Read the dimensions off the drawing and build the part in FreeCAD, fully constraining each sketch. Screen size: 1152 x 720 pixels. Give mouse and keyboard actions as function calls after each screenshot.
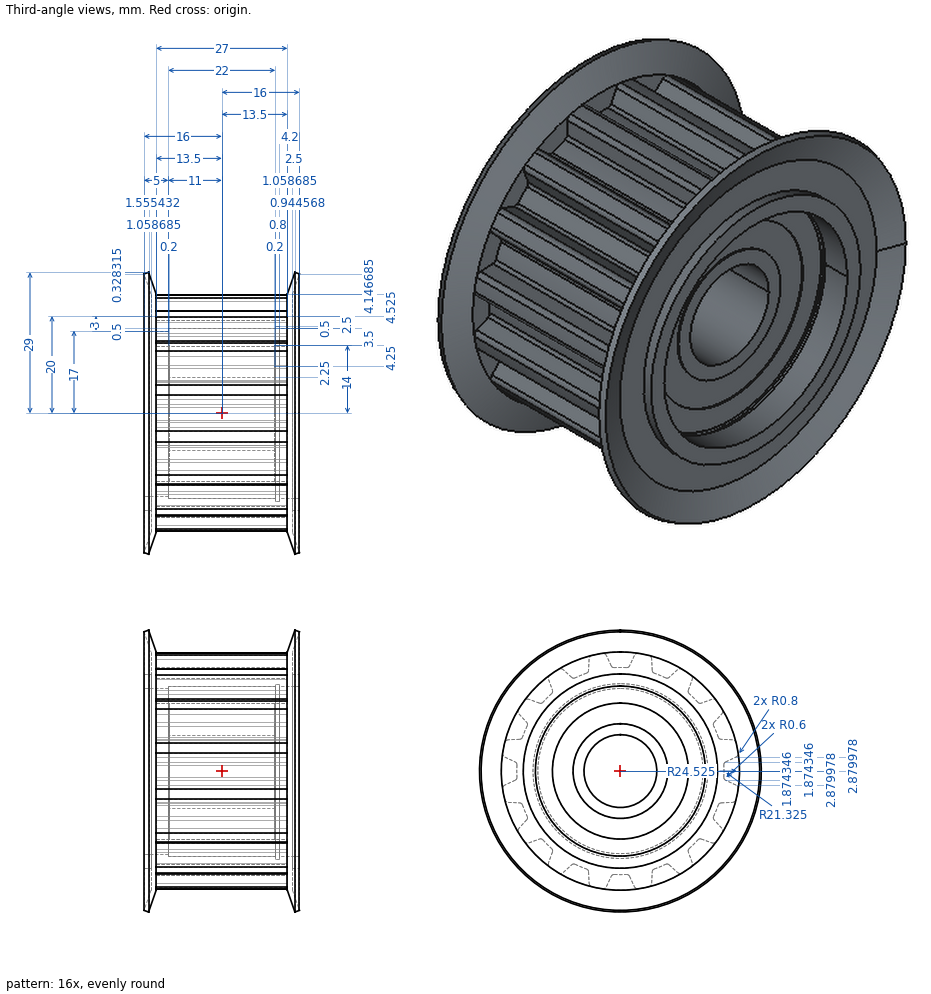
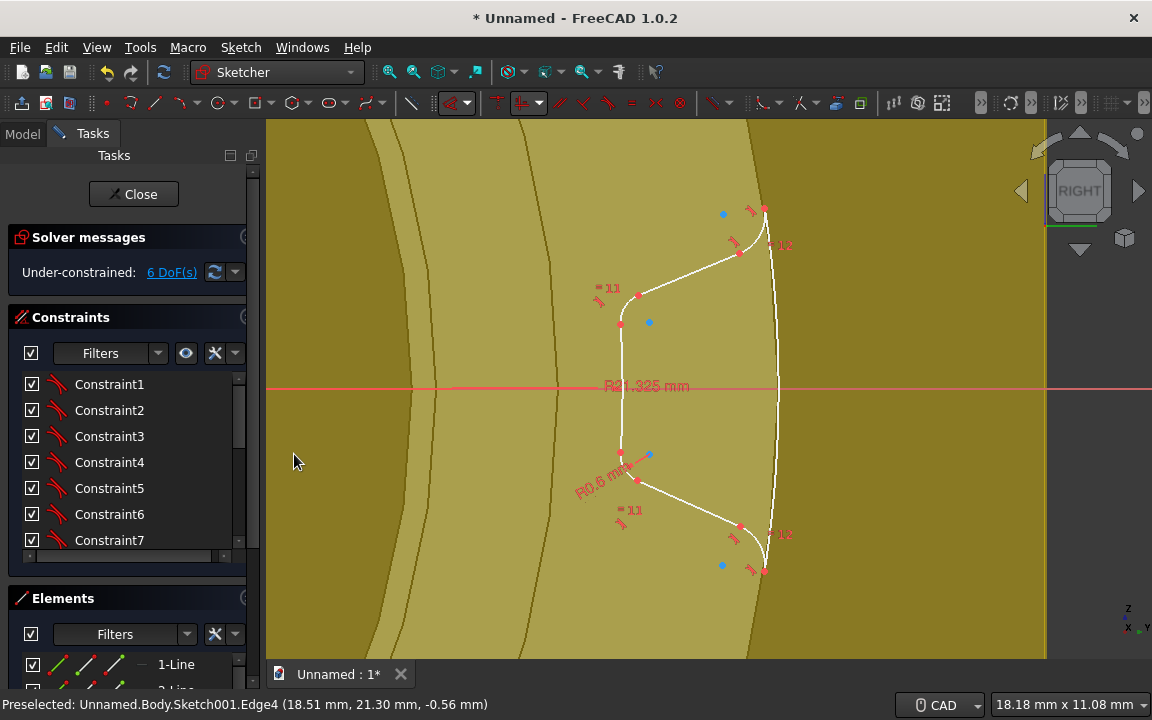
click(753, 244)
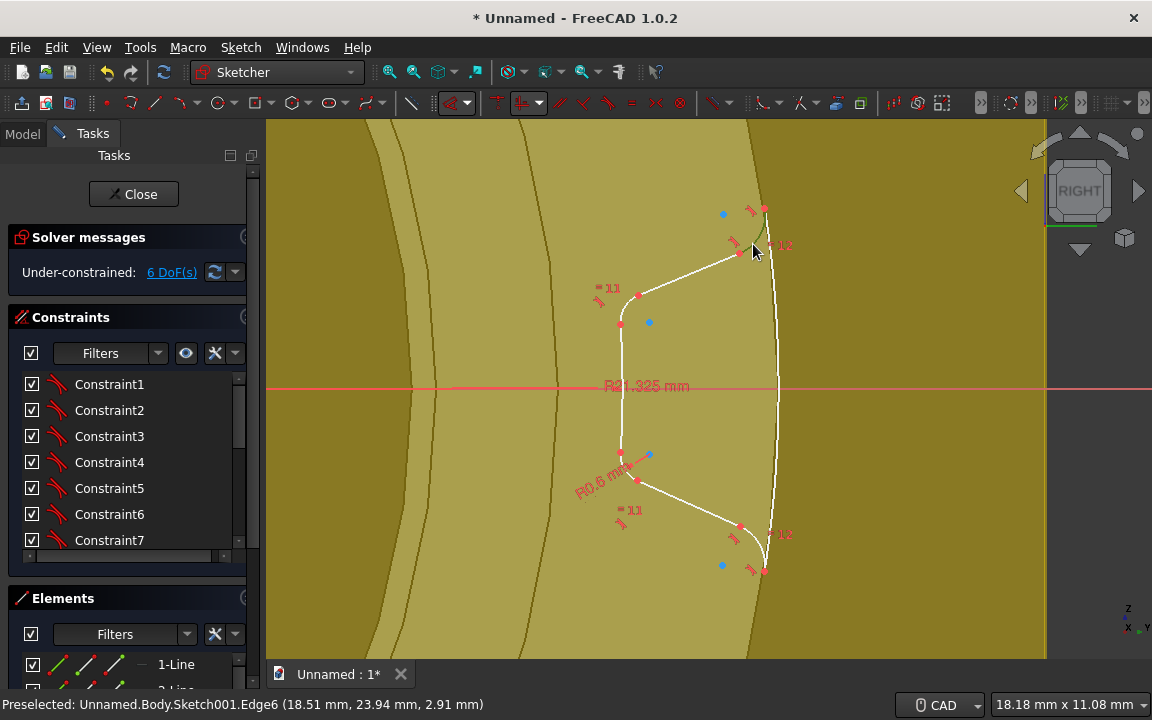
key(k)
key(r)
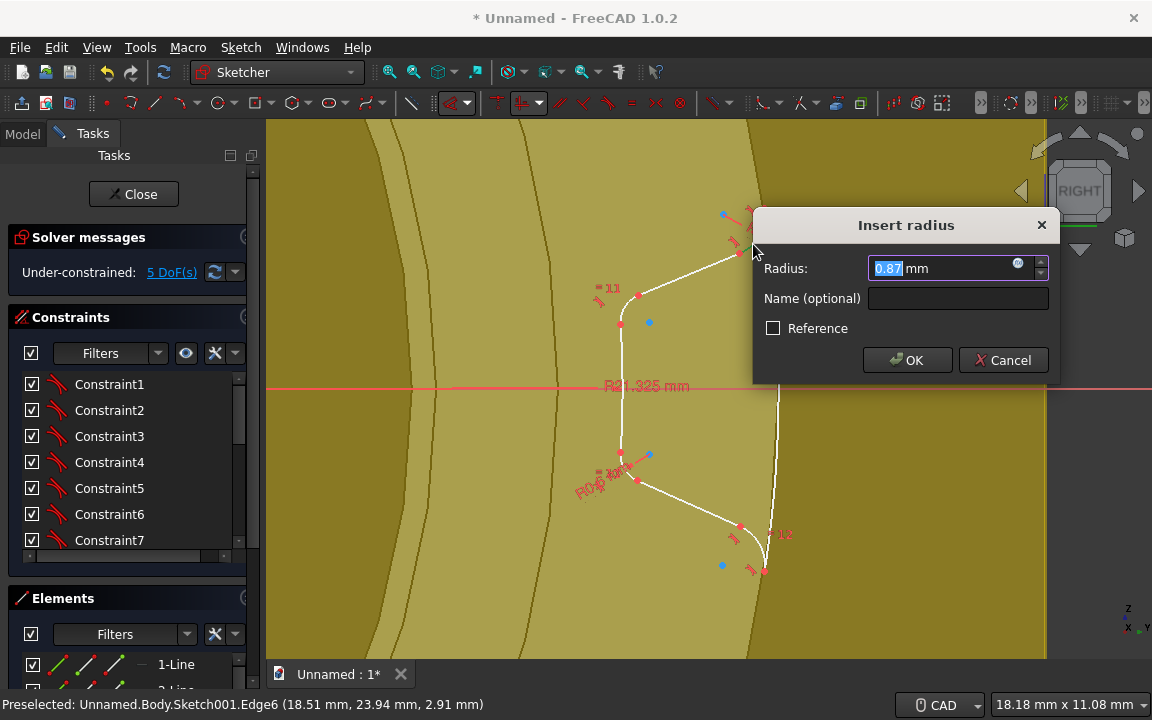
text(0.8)
key(Return)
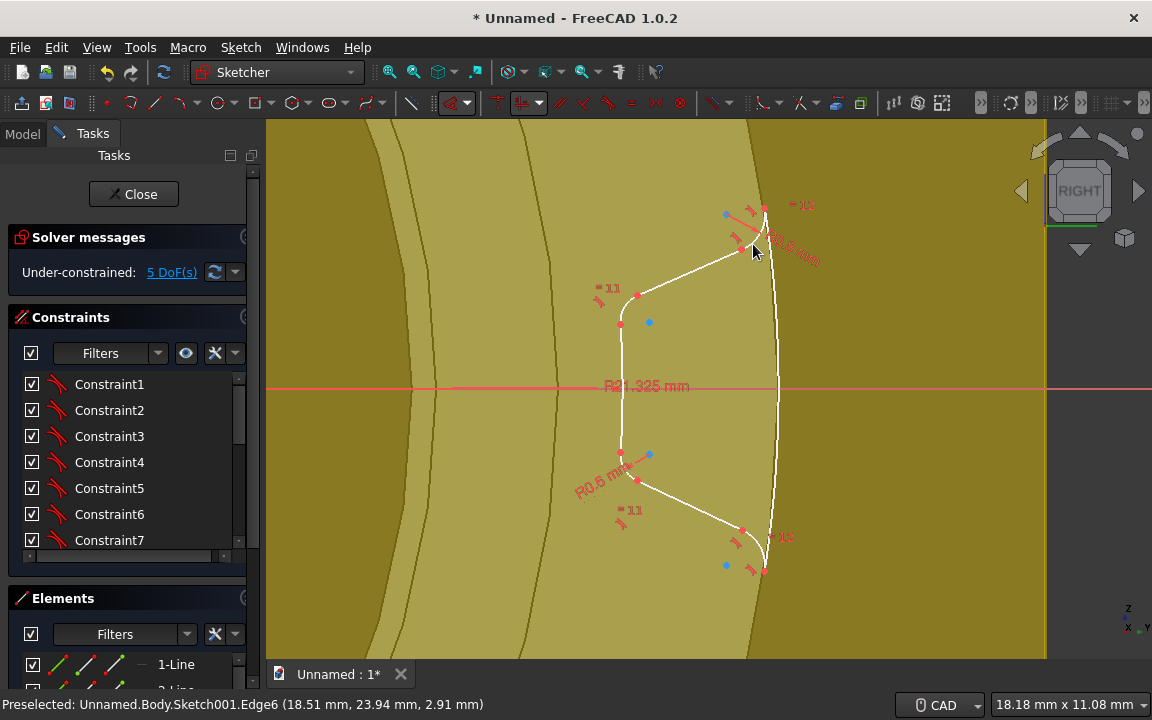
click(776, 463)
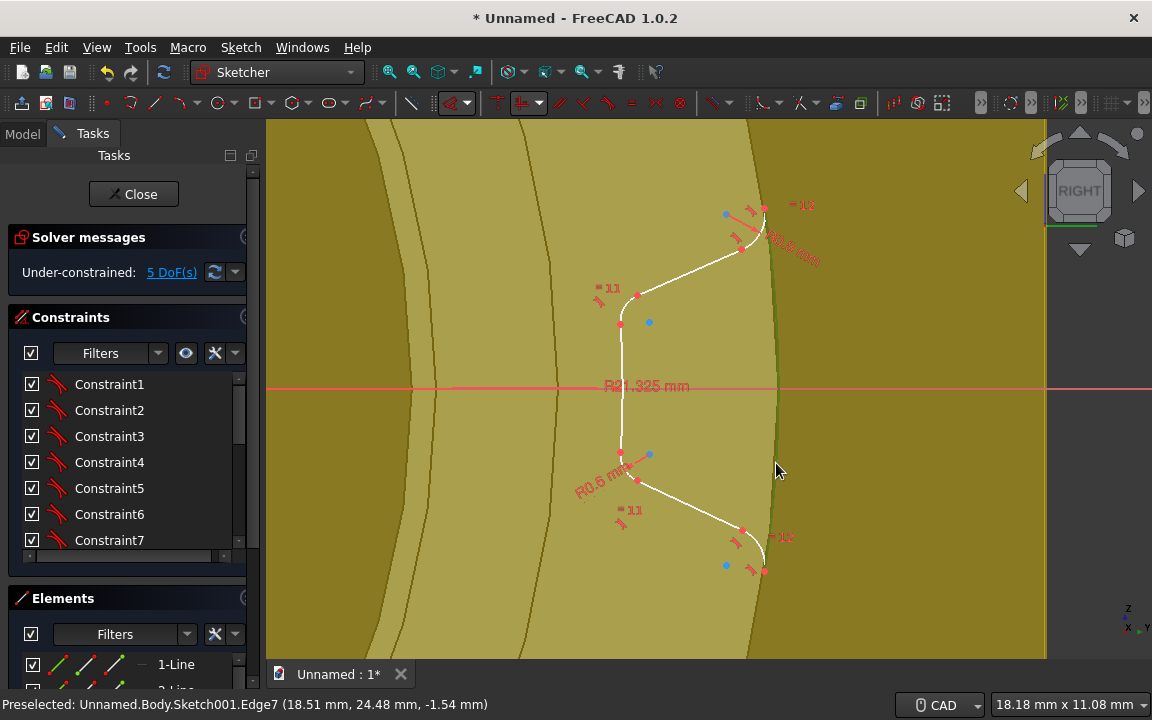
key(k)
key(r)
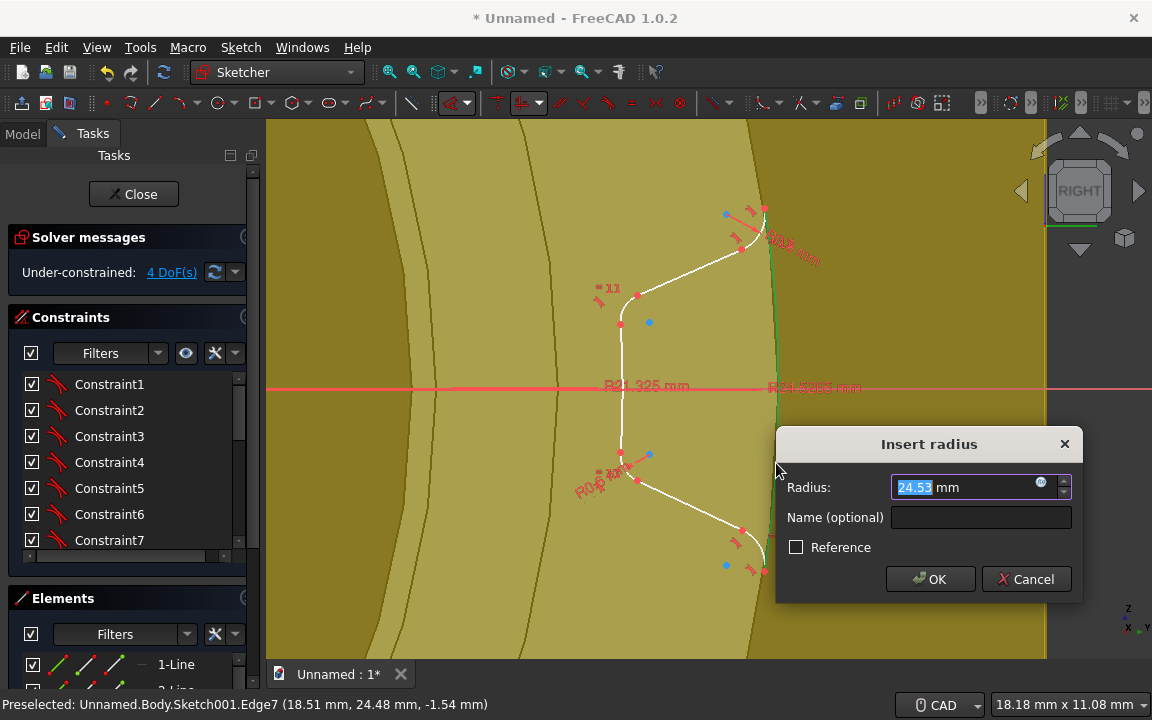
text(24.525)
key(Return)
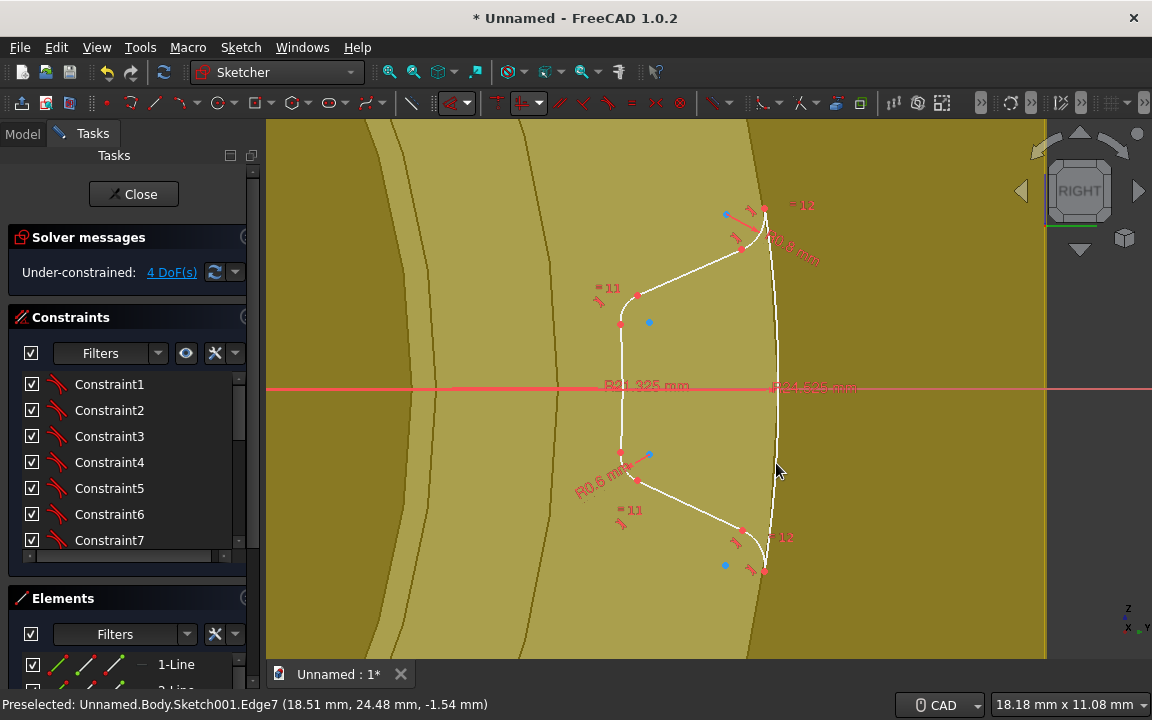
click(743, 530)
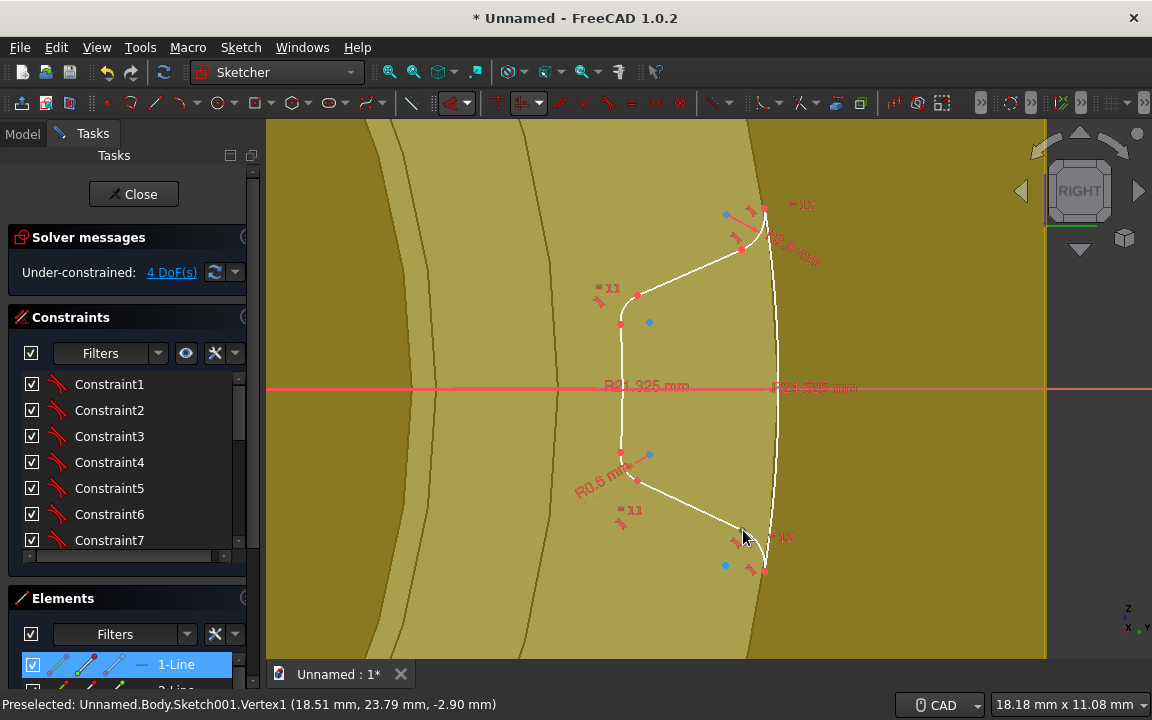
click(470, 104)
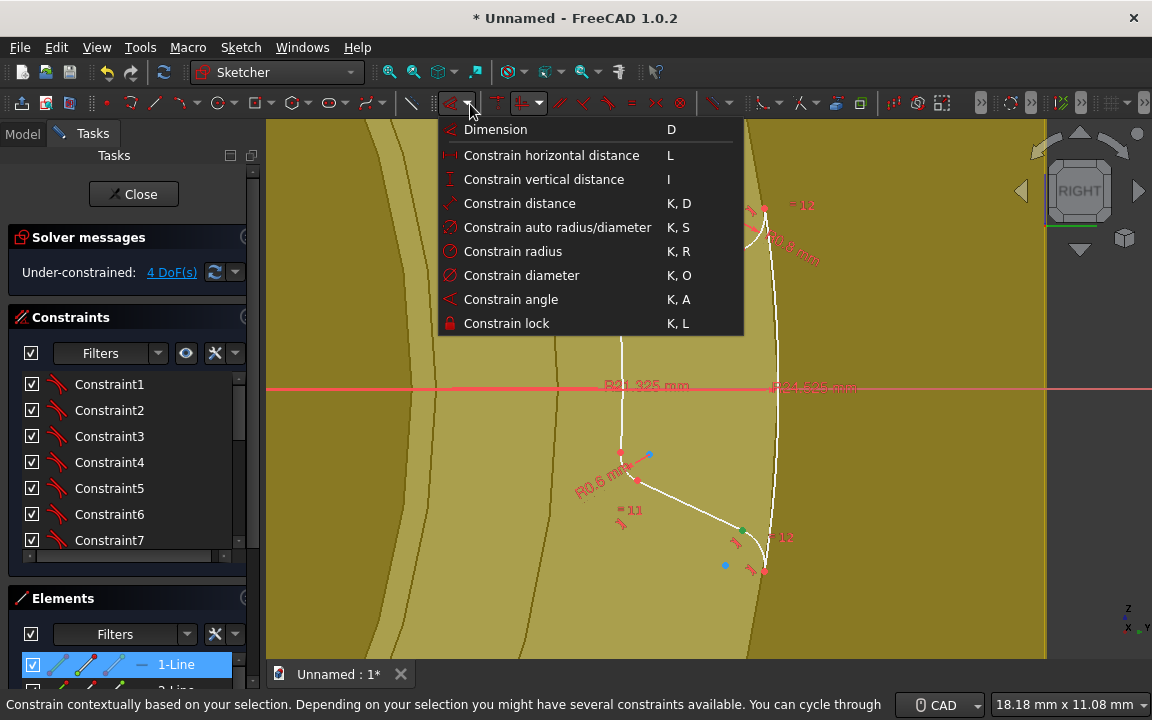
click(591, 179)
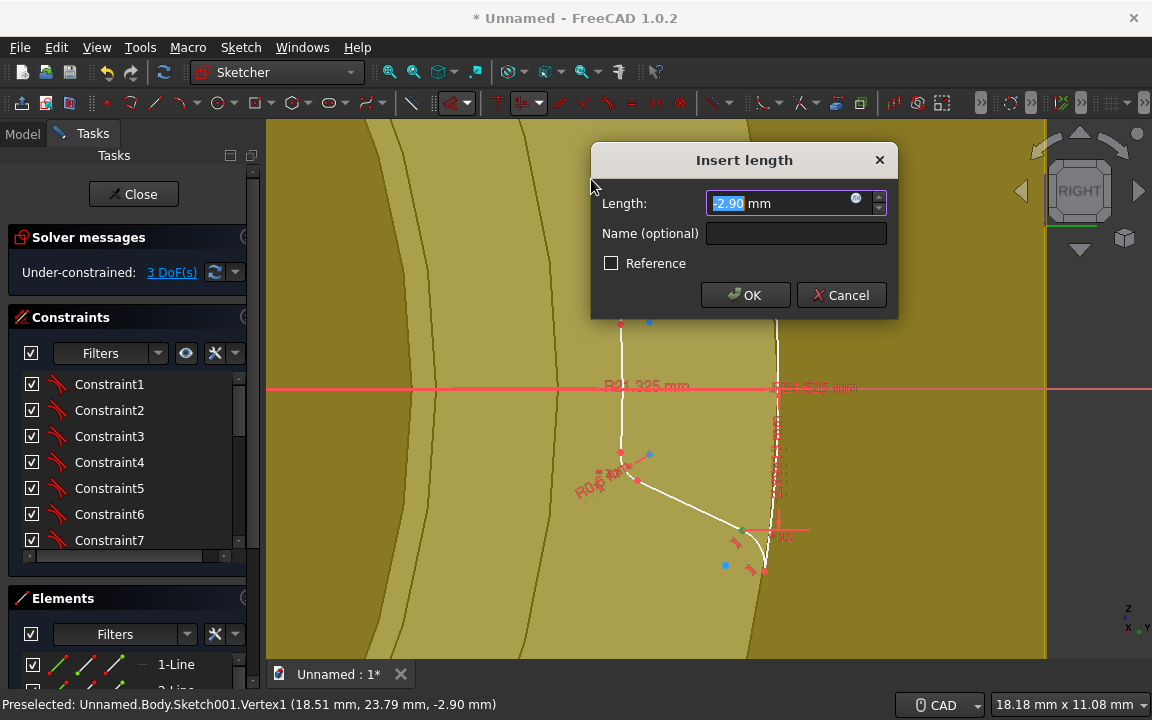
text(-2.879978)
key(Return)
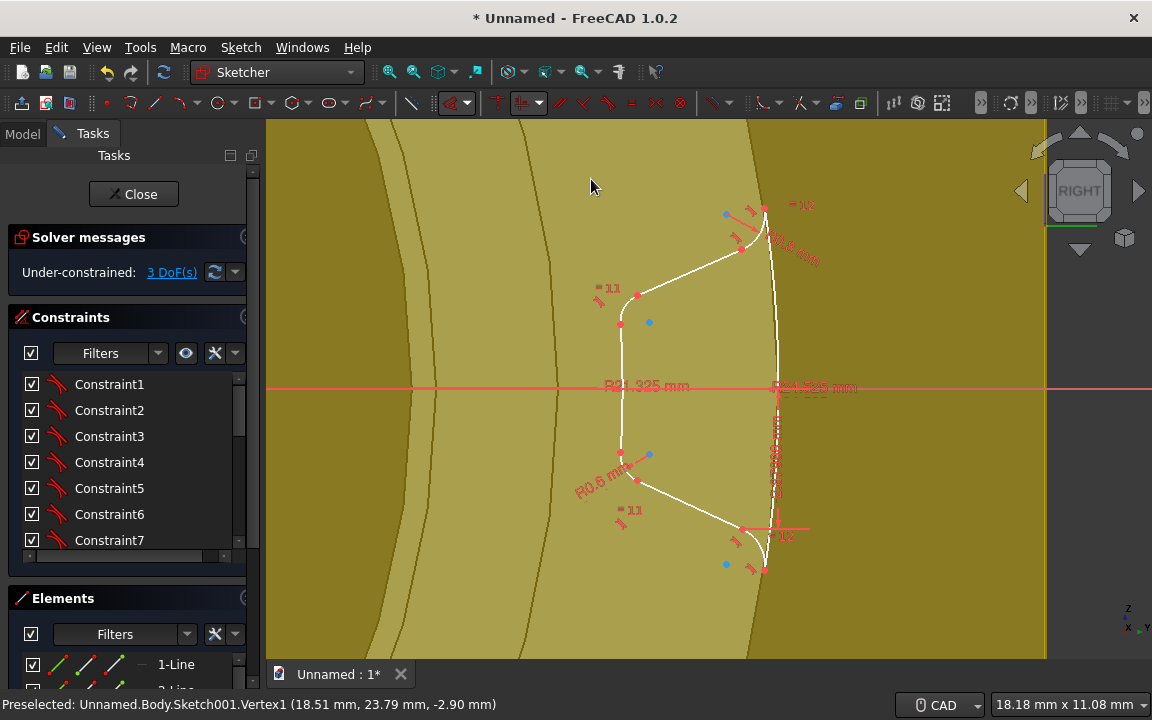
click(638, 481)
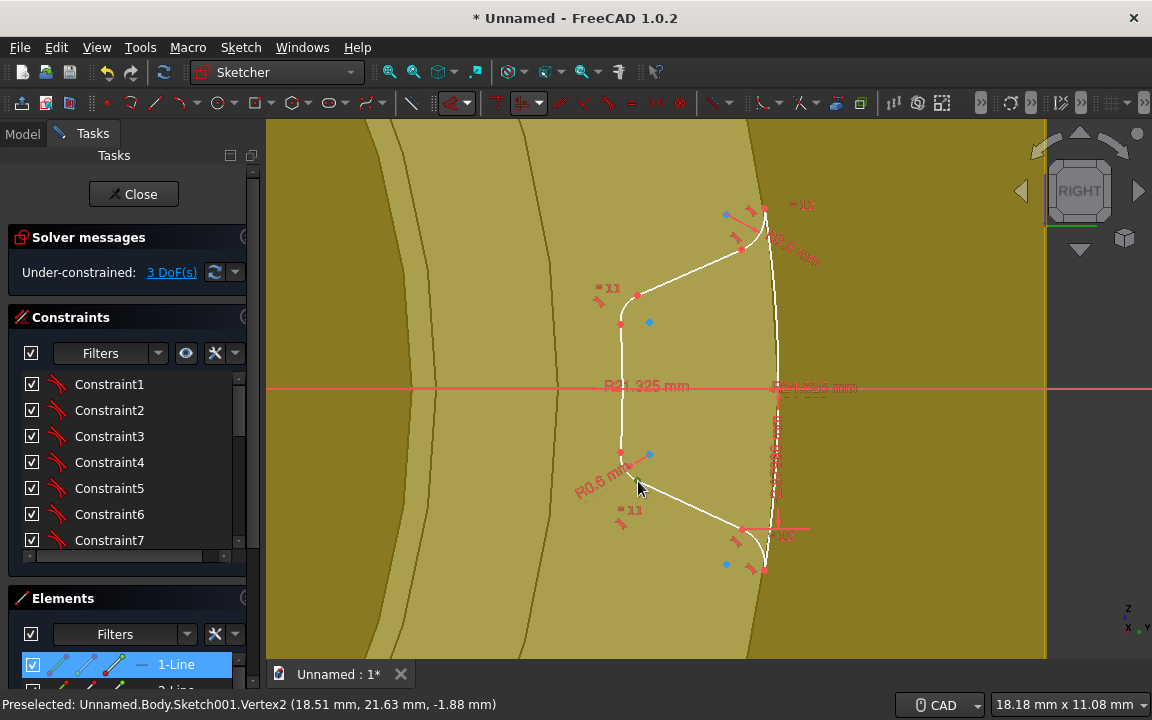
click(470, 104)